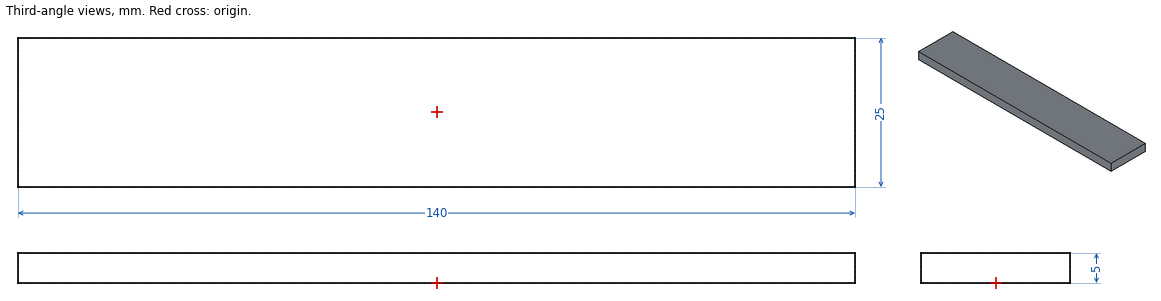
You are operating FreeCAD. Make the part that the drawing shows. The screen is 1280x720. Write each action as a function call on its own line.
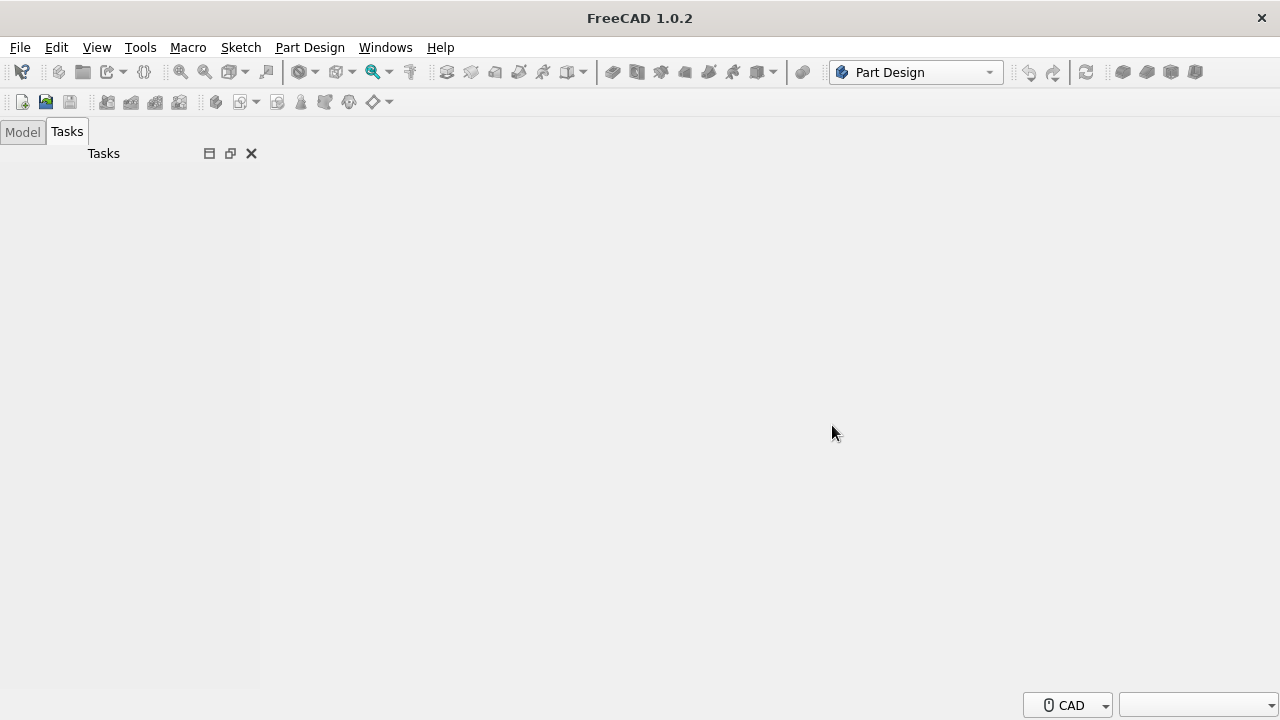
click(22, 102)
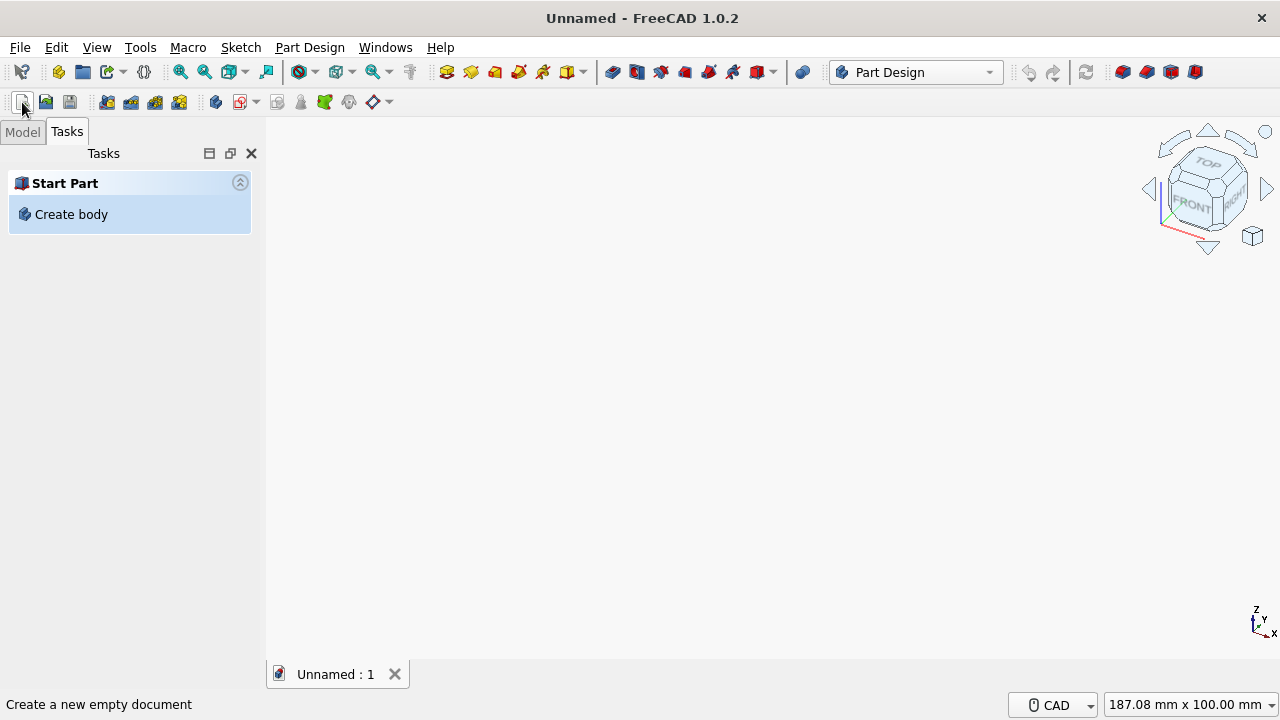
click(240, 102)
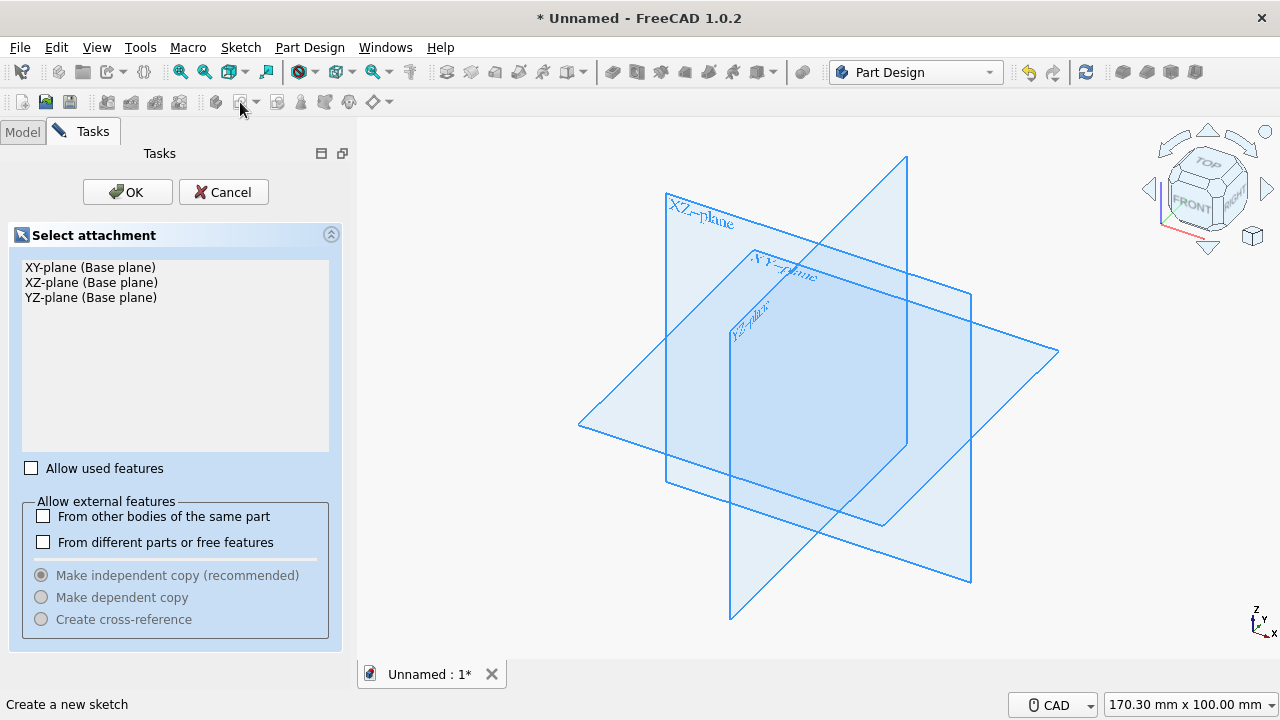
click(82, 268)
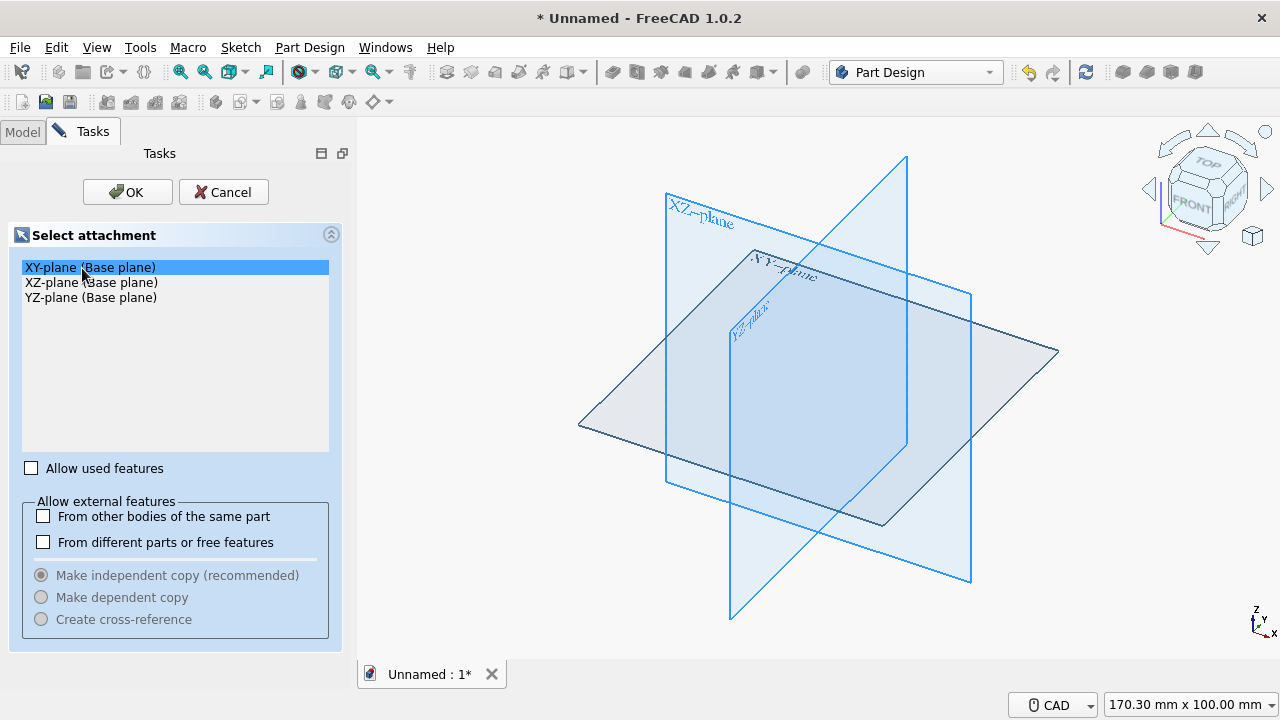
click(128, 192)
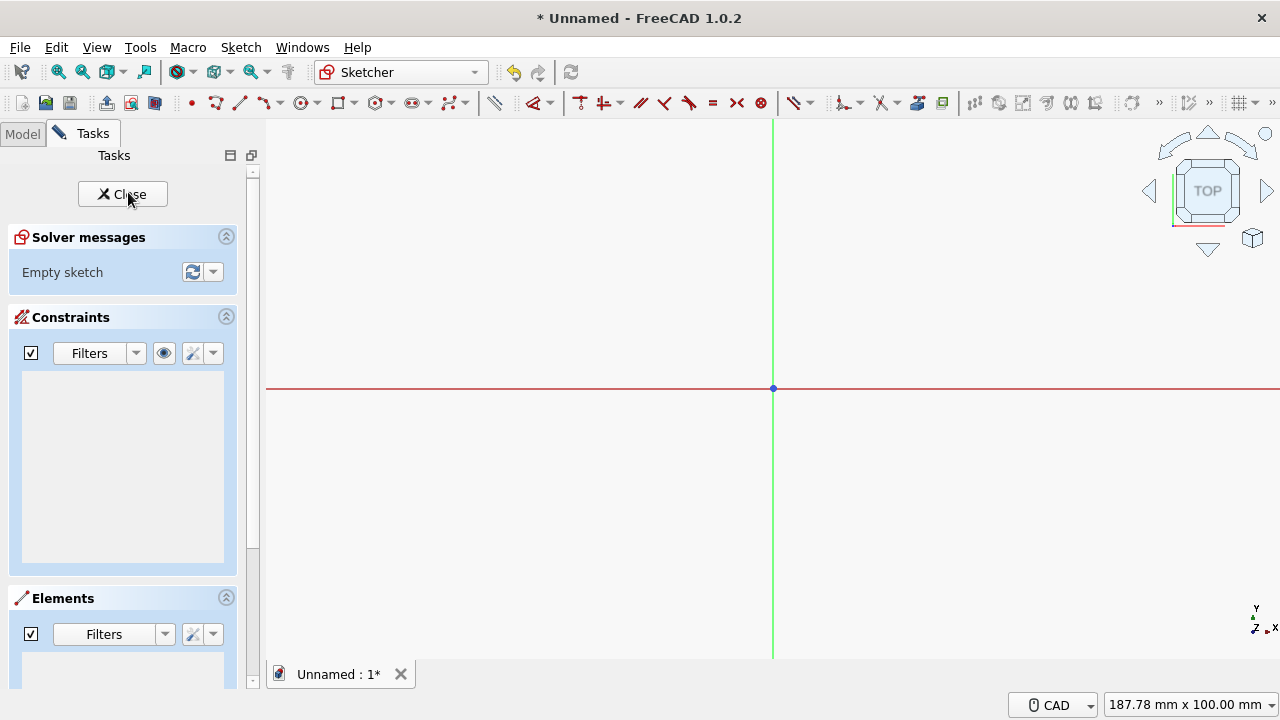
scroll(395, 389, down, 1)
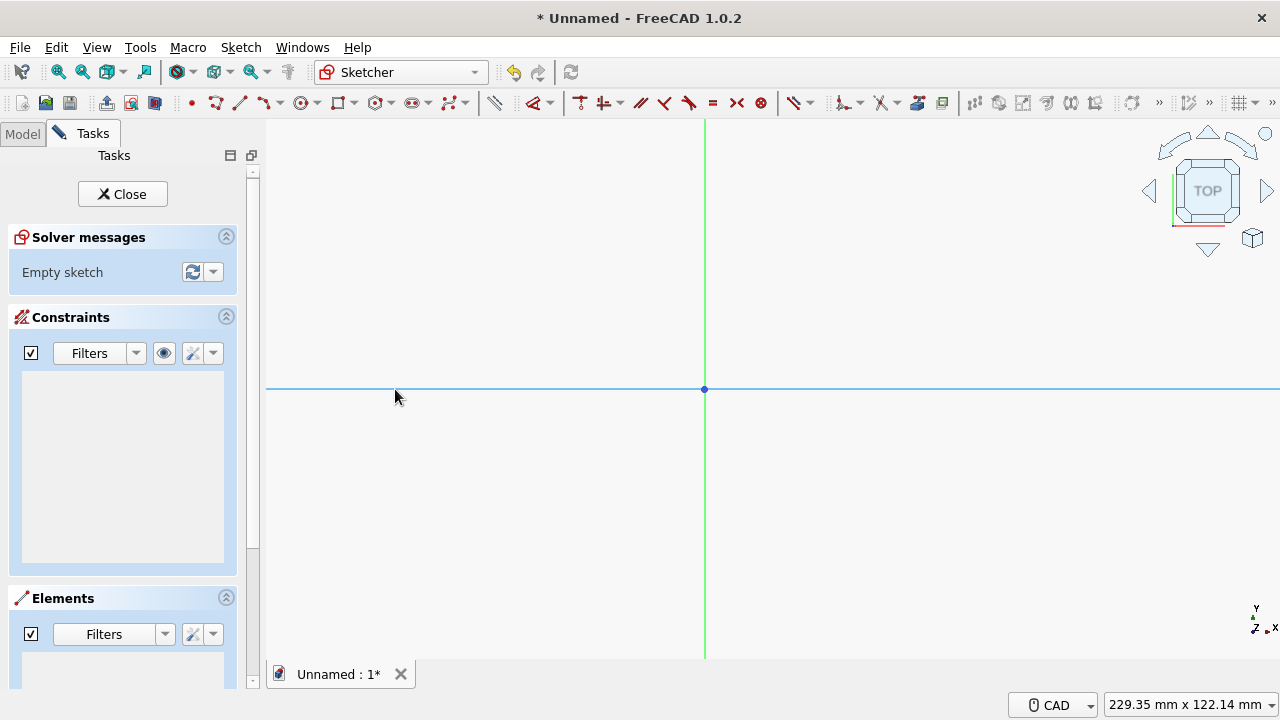
click(356, 104)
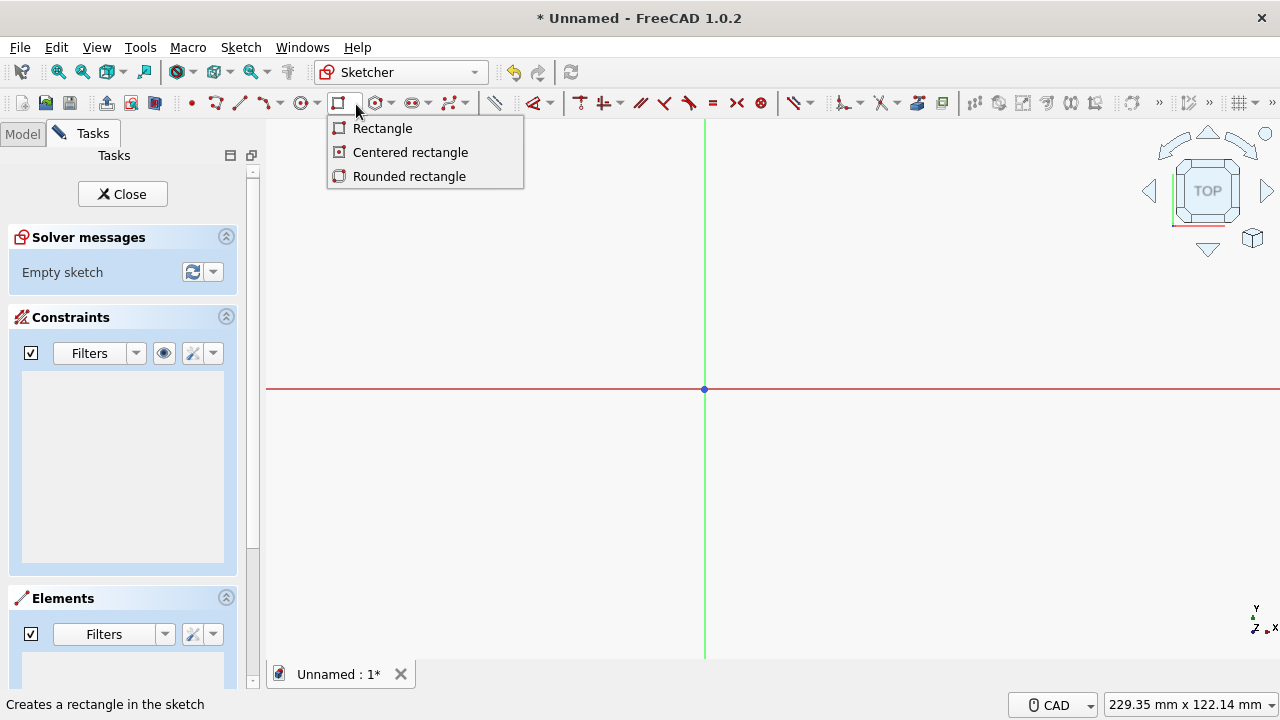
click(426, 152)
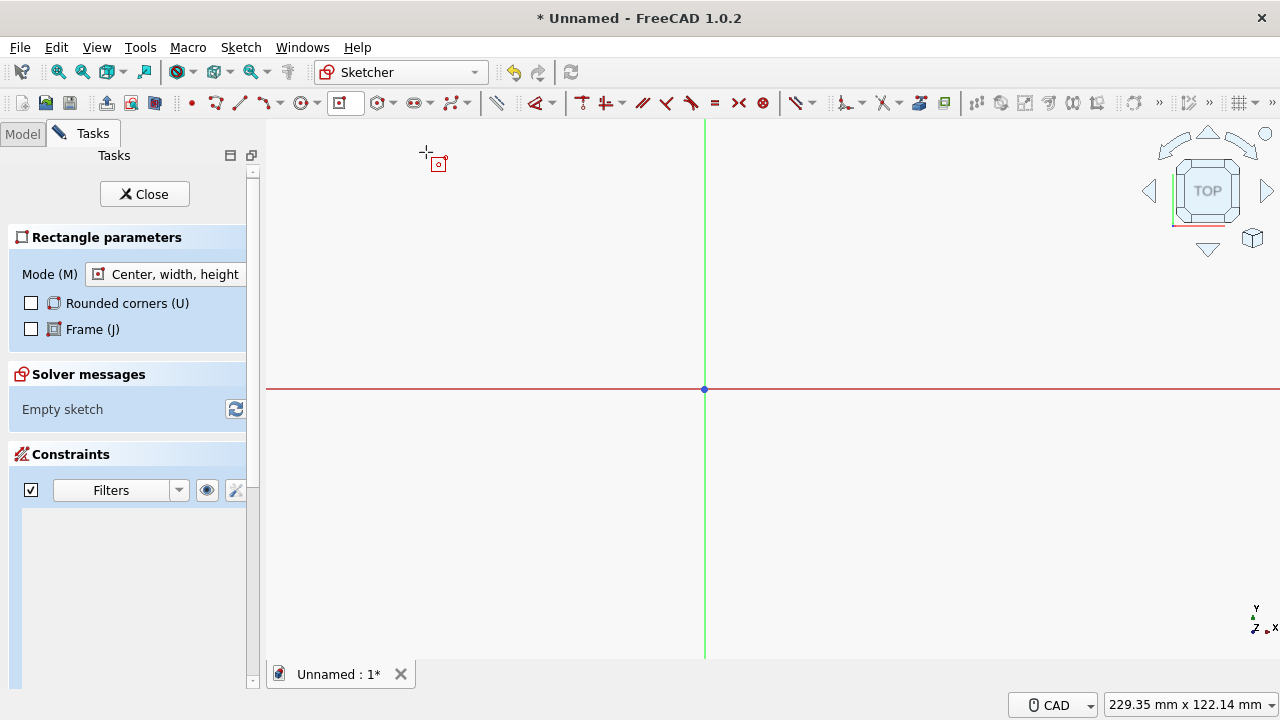
click(705, 389)
click(1014, 334)
key(Escape)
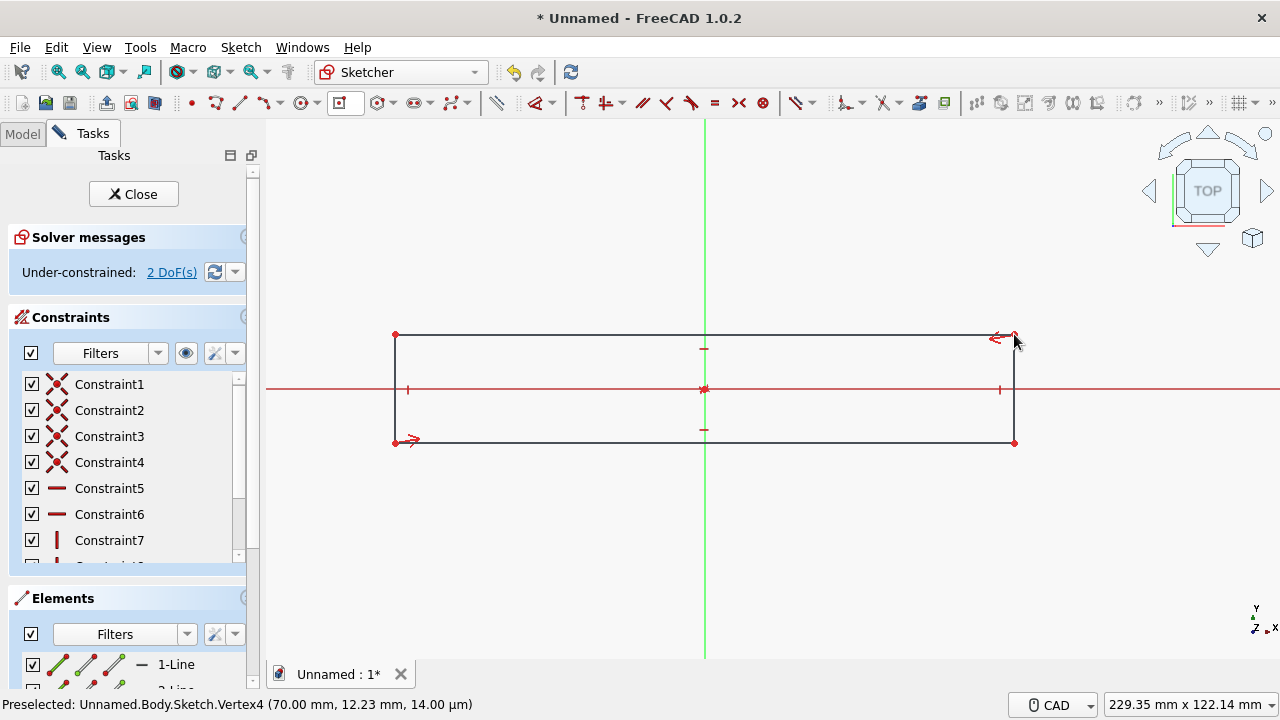
key(d)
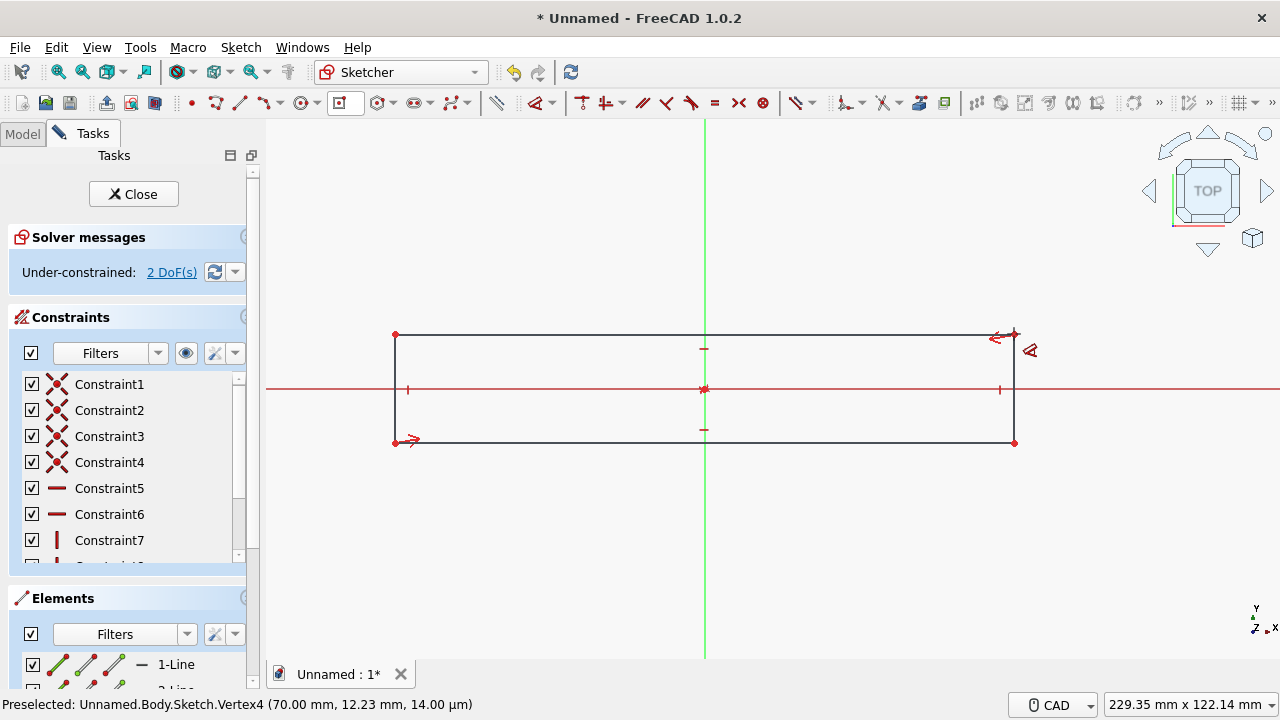
click(1014, 411)
click(1048, 364)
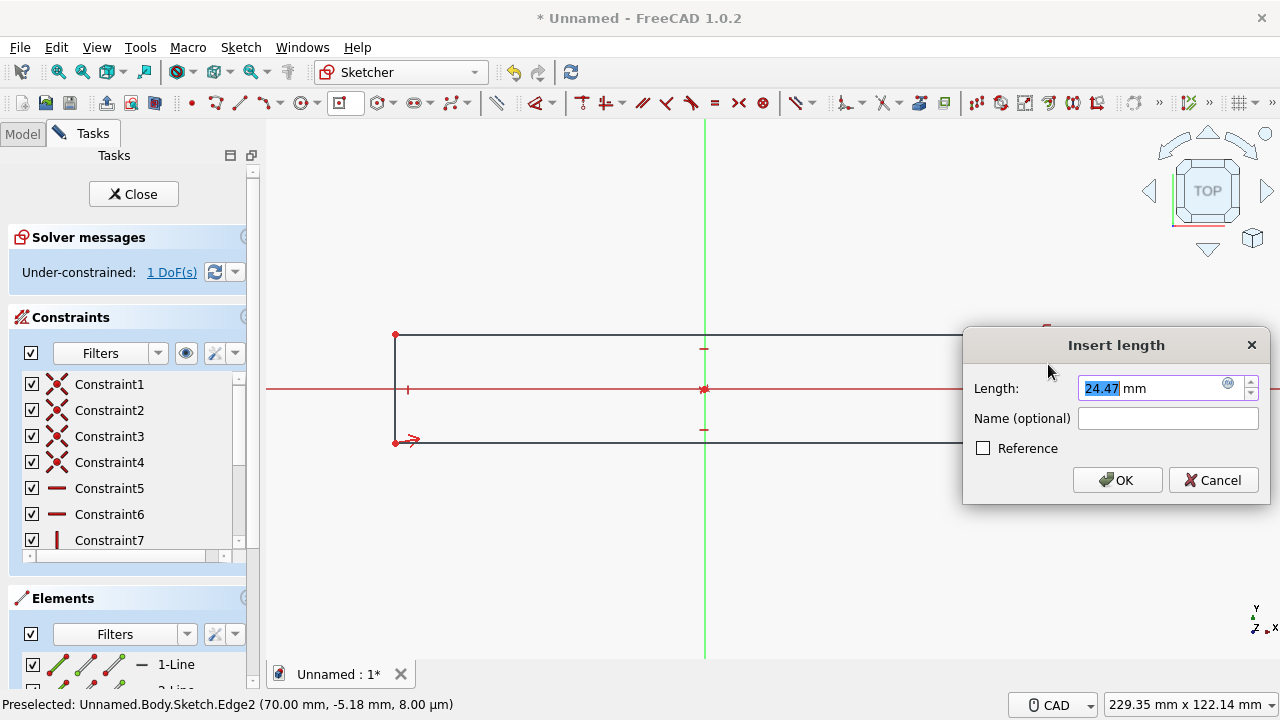
text(25)
key(Return)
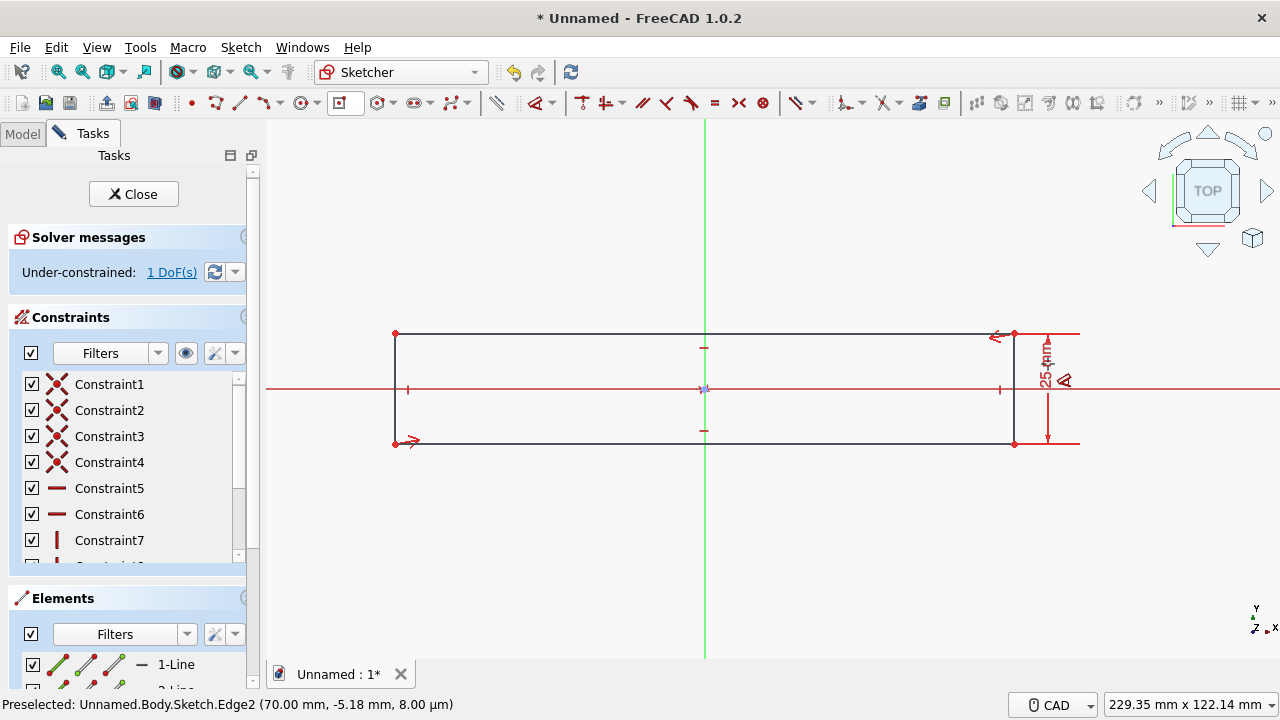
click(581, 444)
click(562, 478)